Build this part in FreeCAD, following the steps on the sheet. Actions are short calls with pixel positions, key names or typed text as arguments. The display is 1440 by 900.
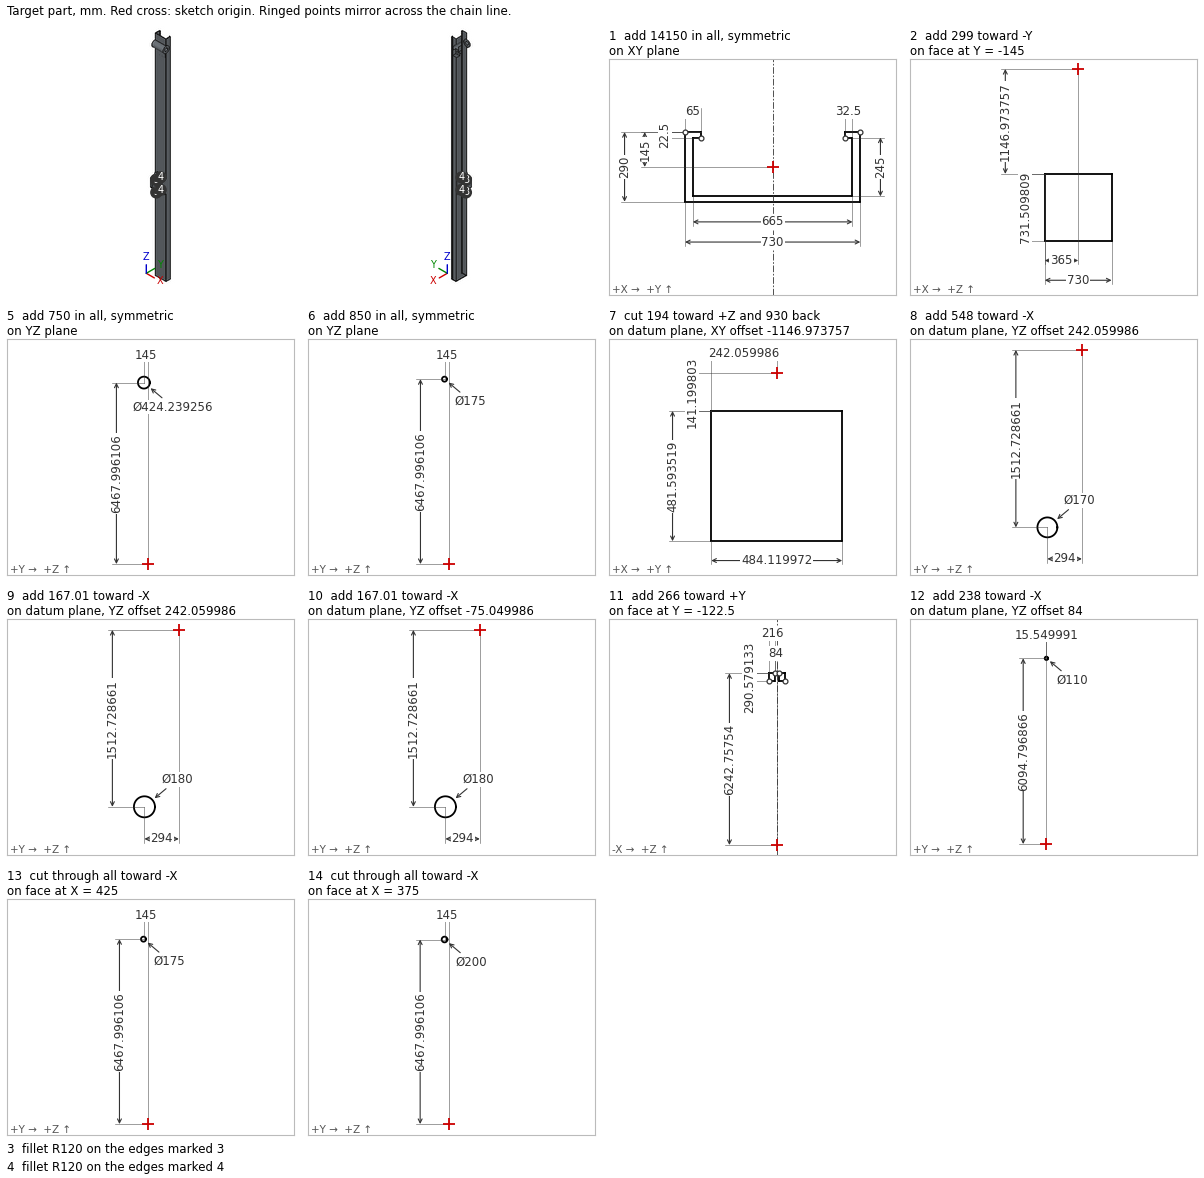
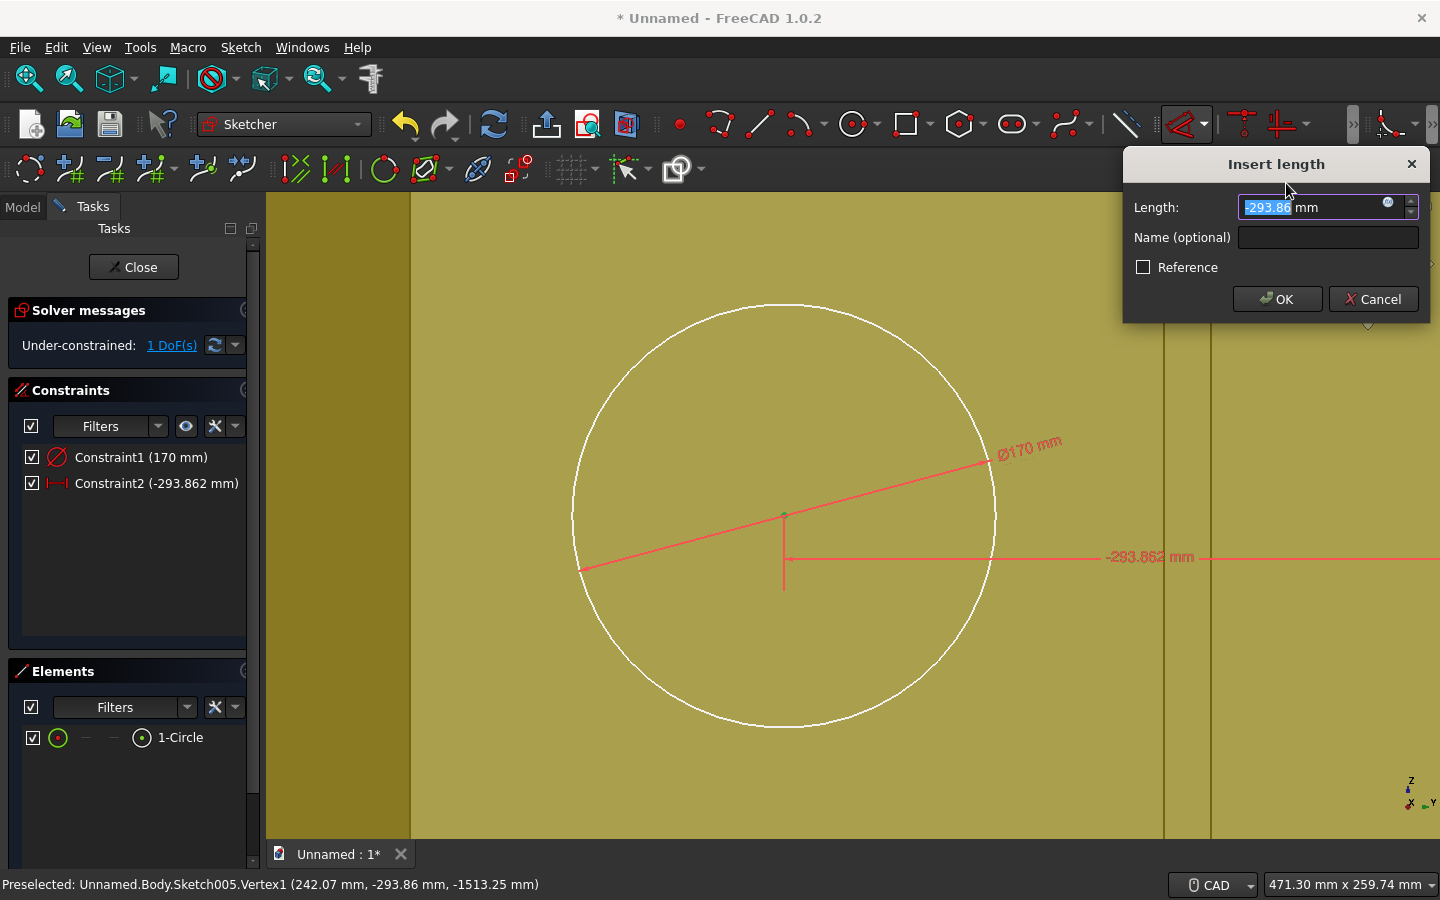
text(-294)
key(Return)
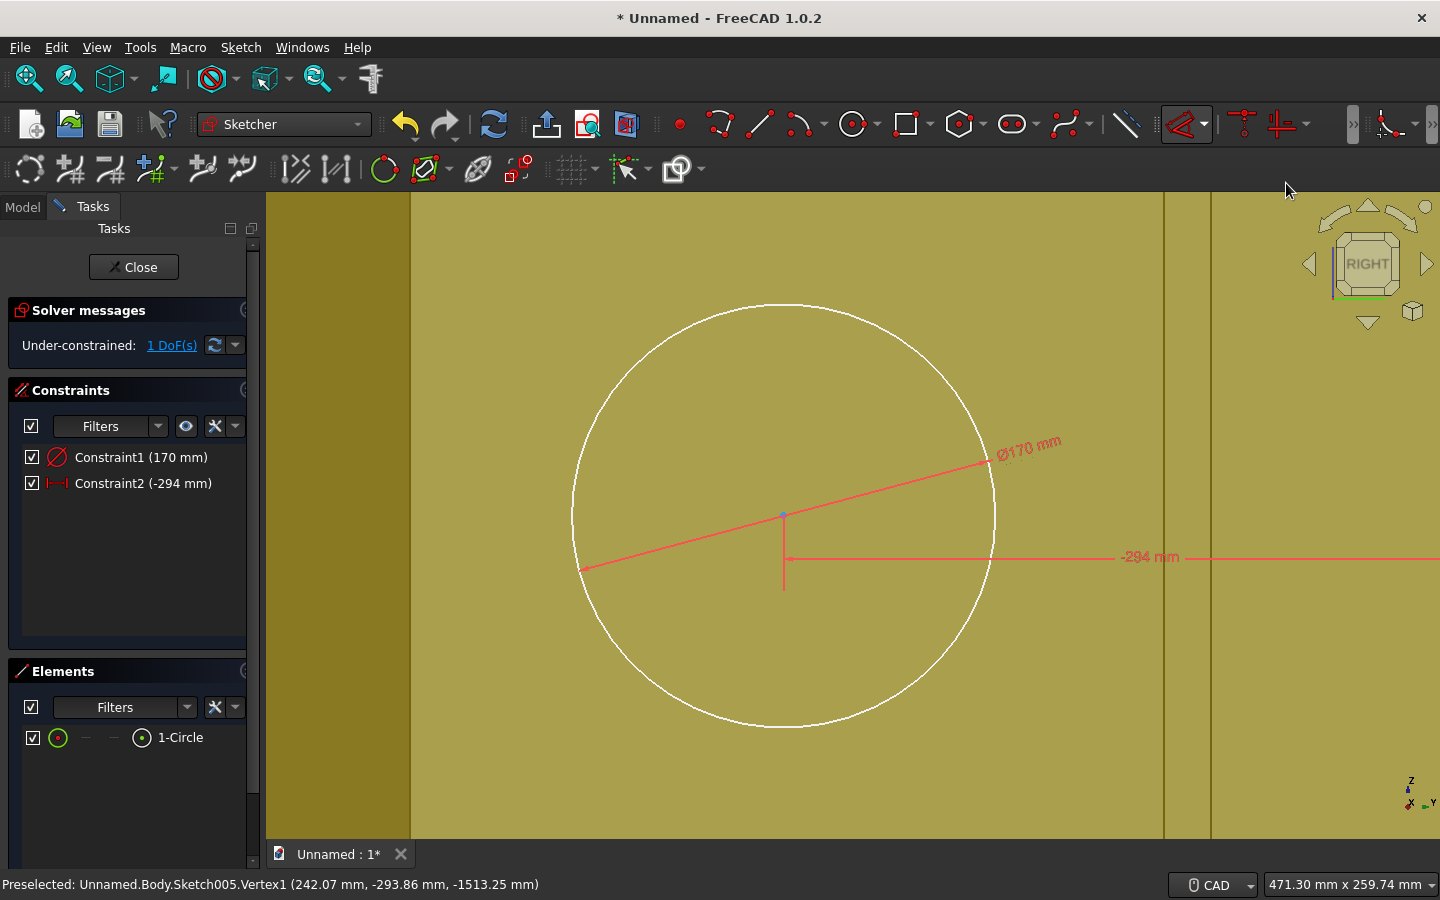
click(784, 516)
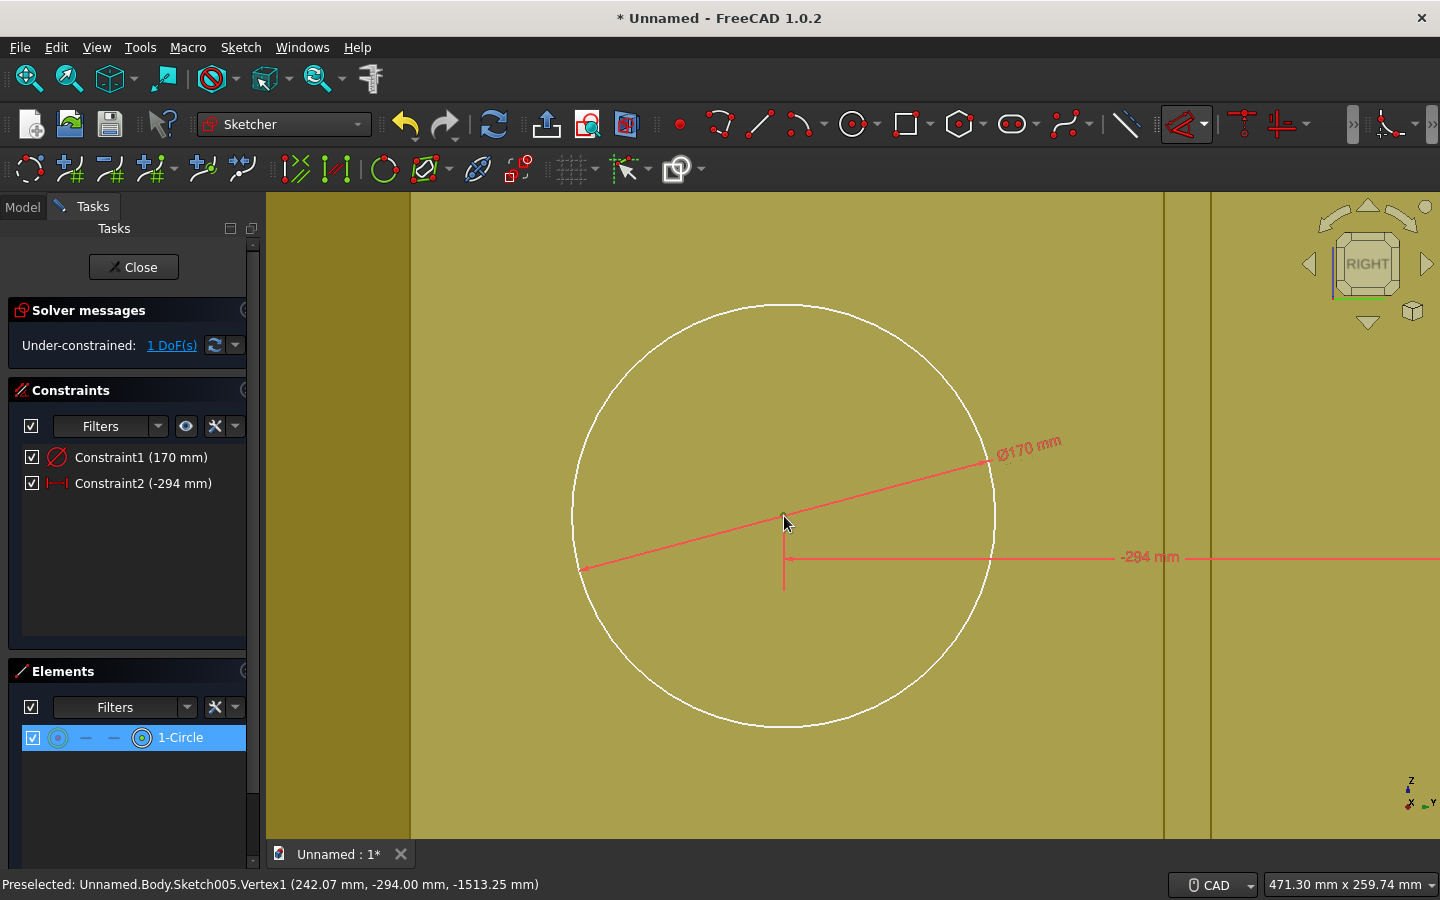
click(1206, 124)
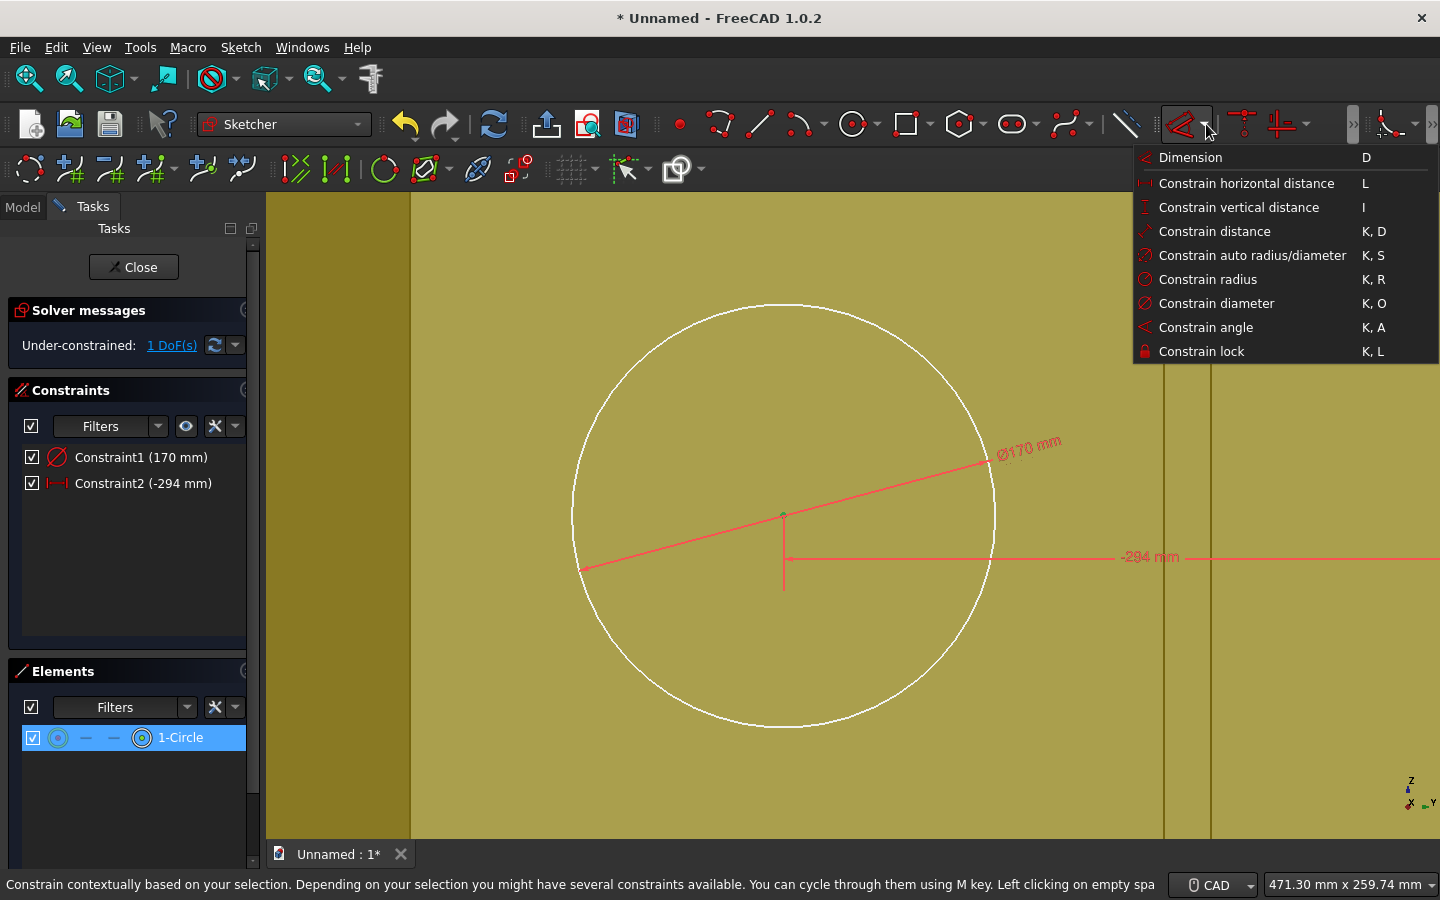
click(1286, 207)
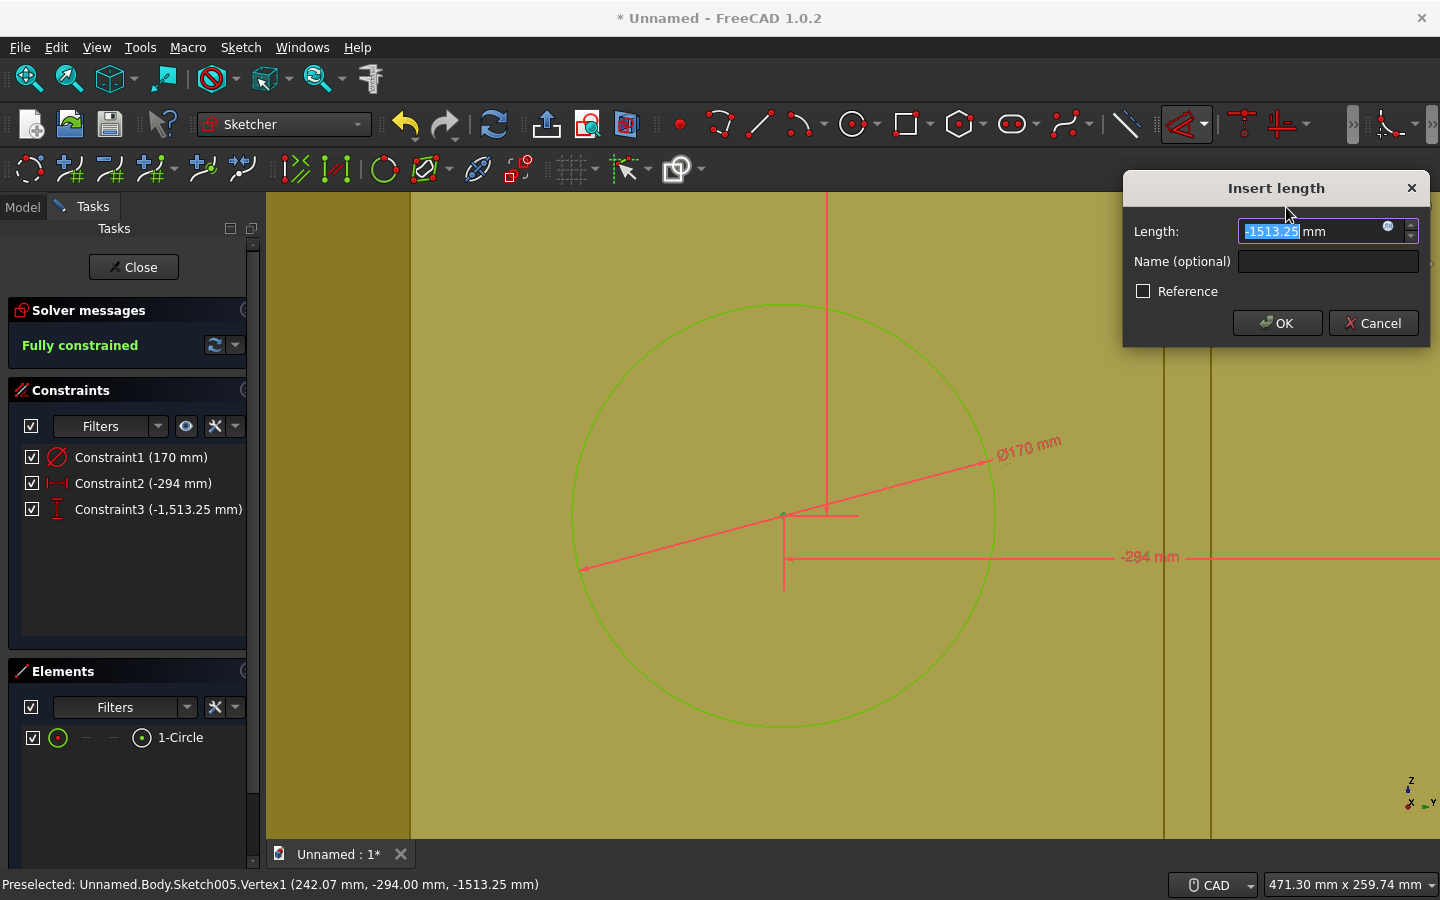
text(-1512.728661)
key(Return)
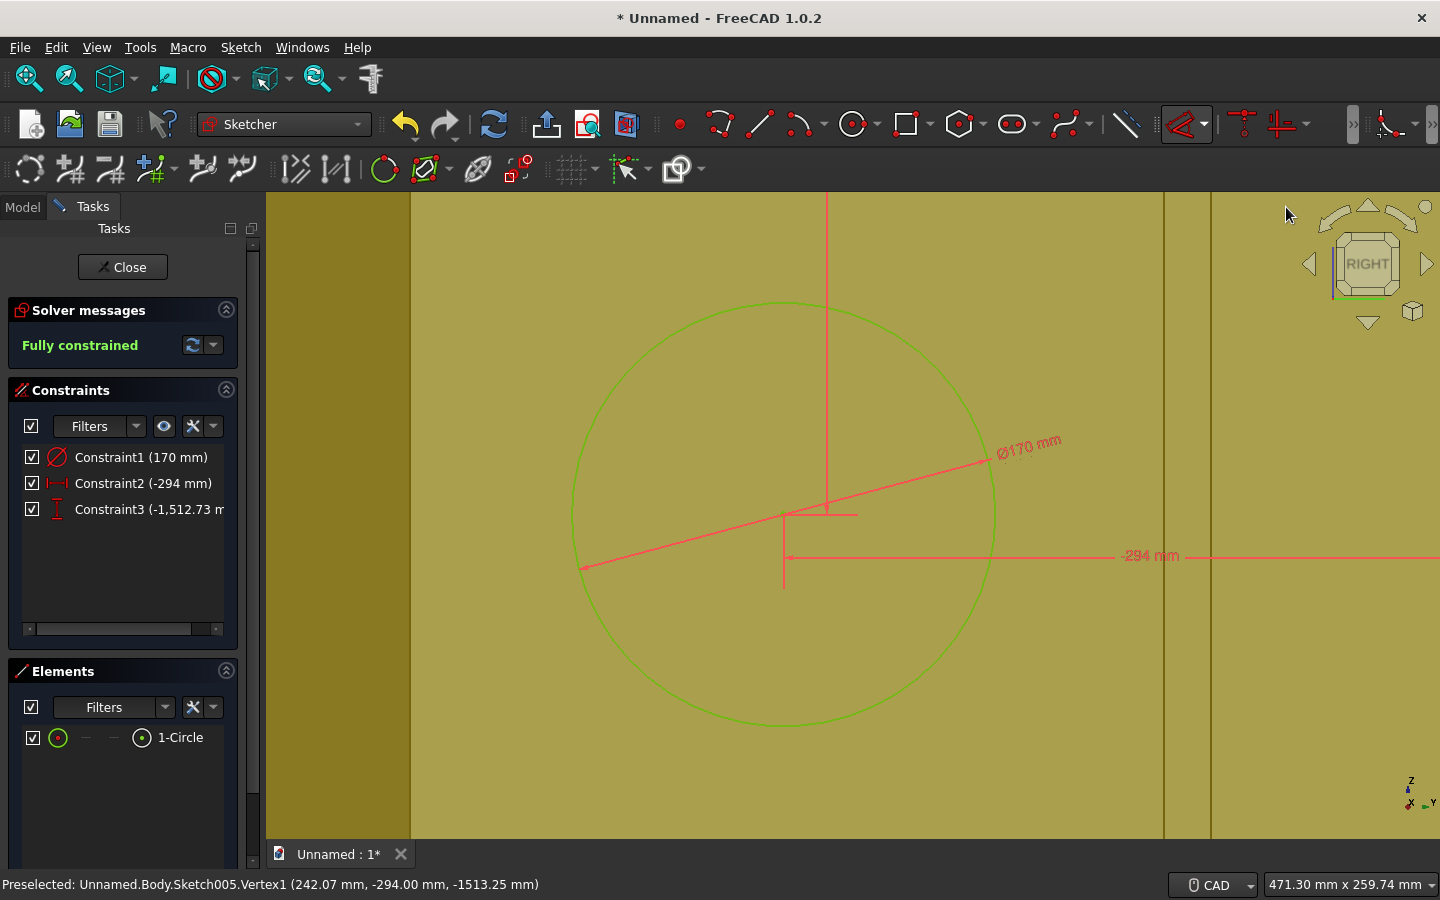
click(123, 267)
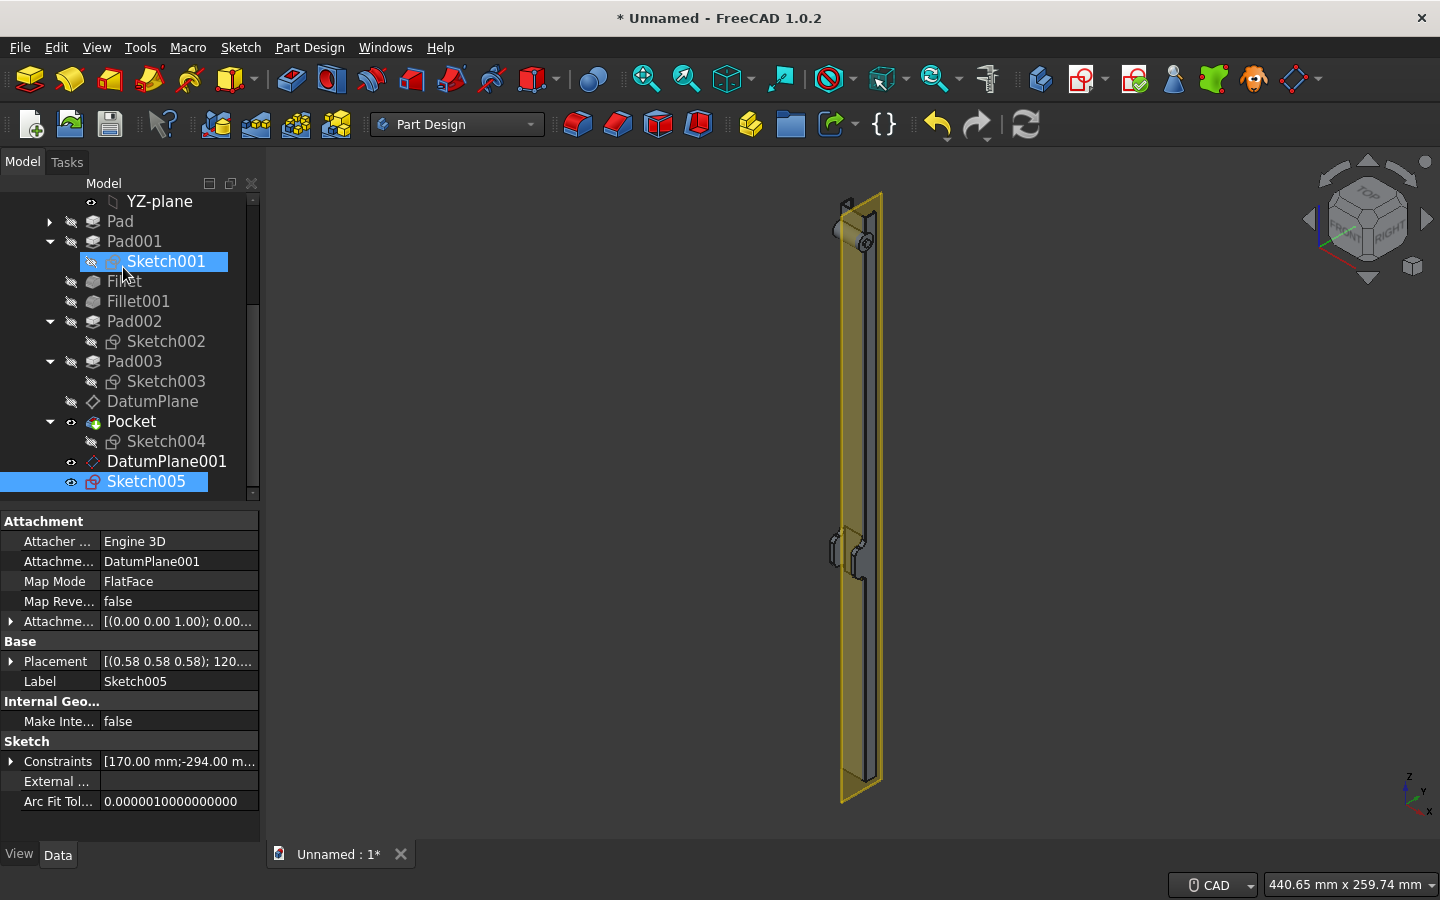
click(30, 80)